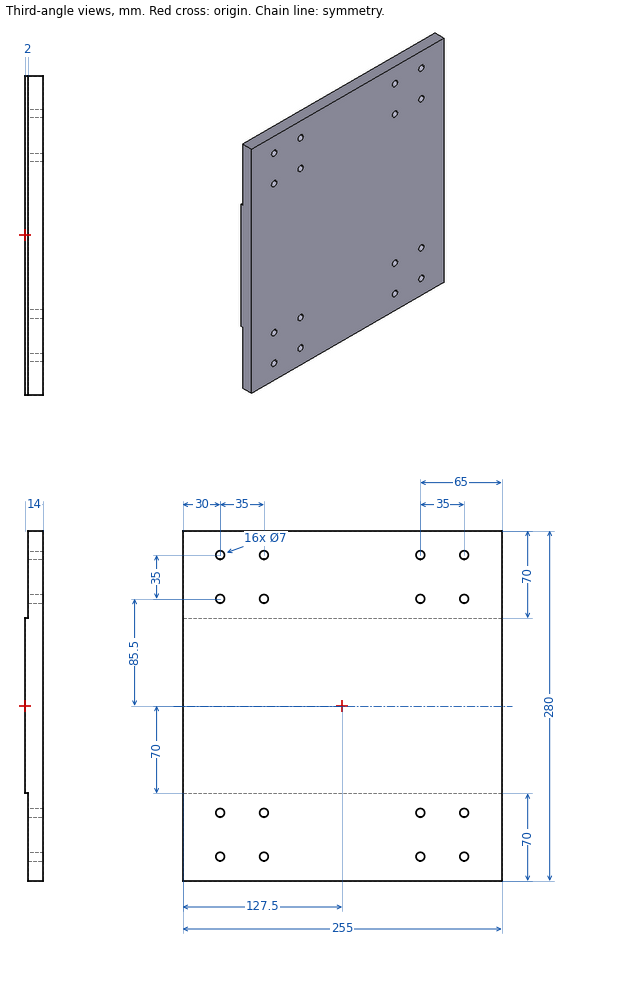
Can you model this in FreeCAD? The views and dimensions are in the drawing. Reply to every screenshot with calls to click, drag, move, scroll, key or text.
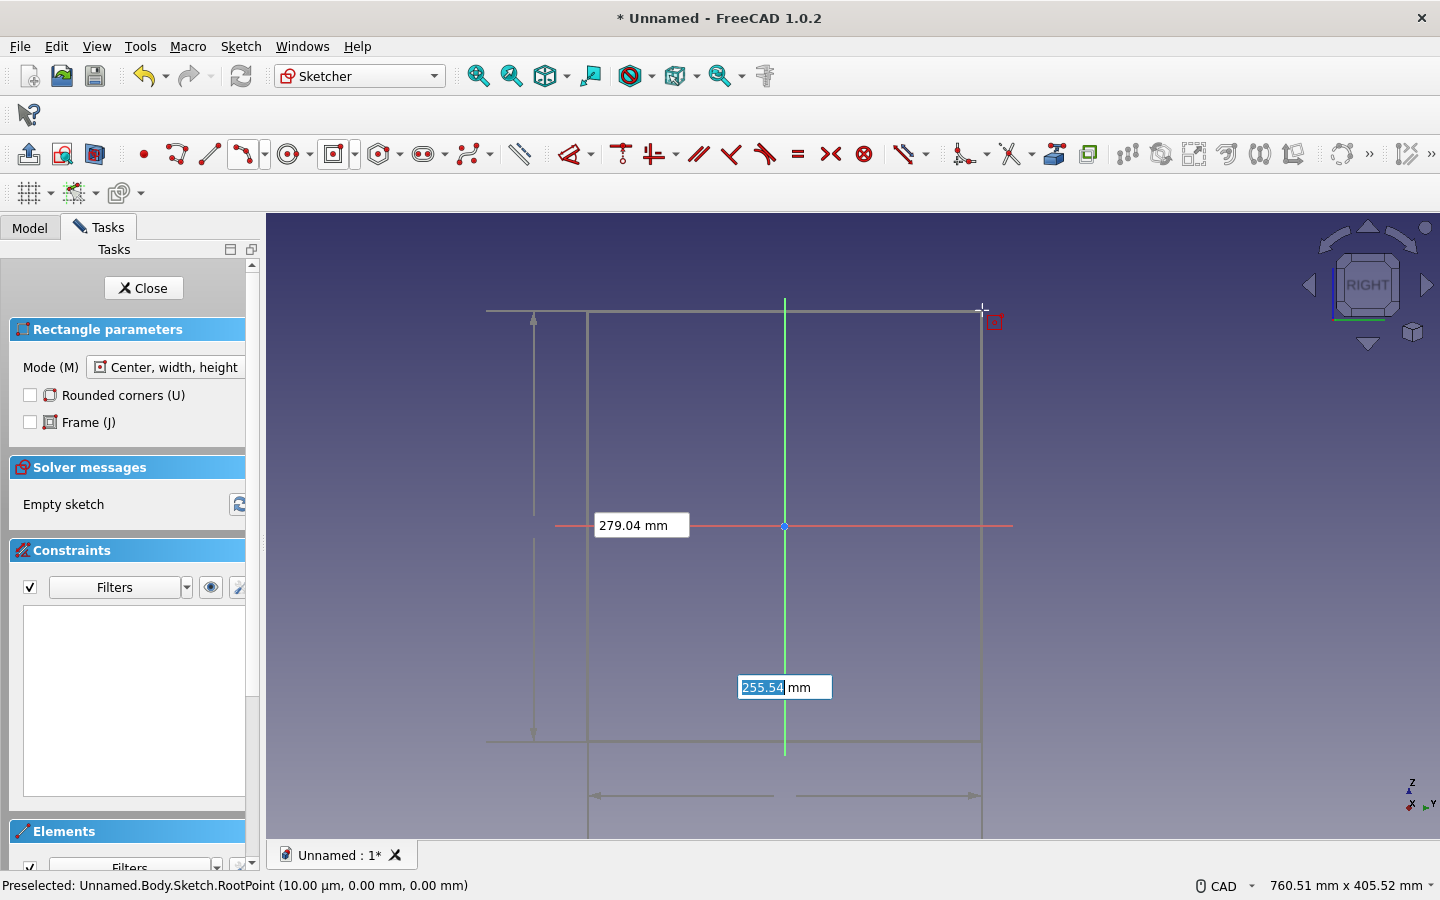
text(255)
key(Tab)
text(280)
key(Return)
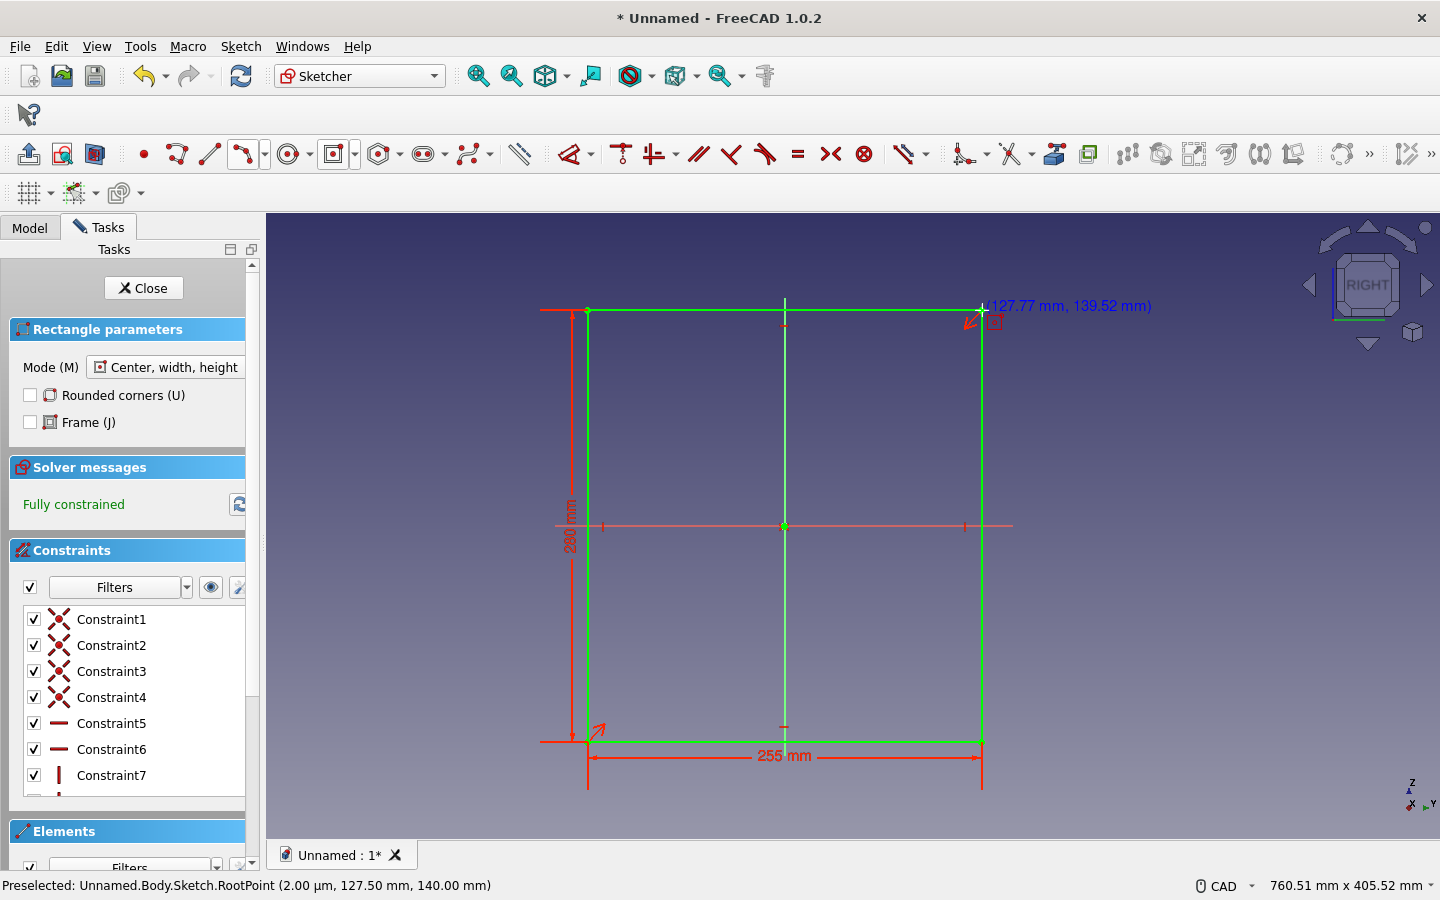
click(288, 154)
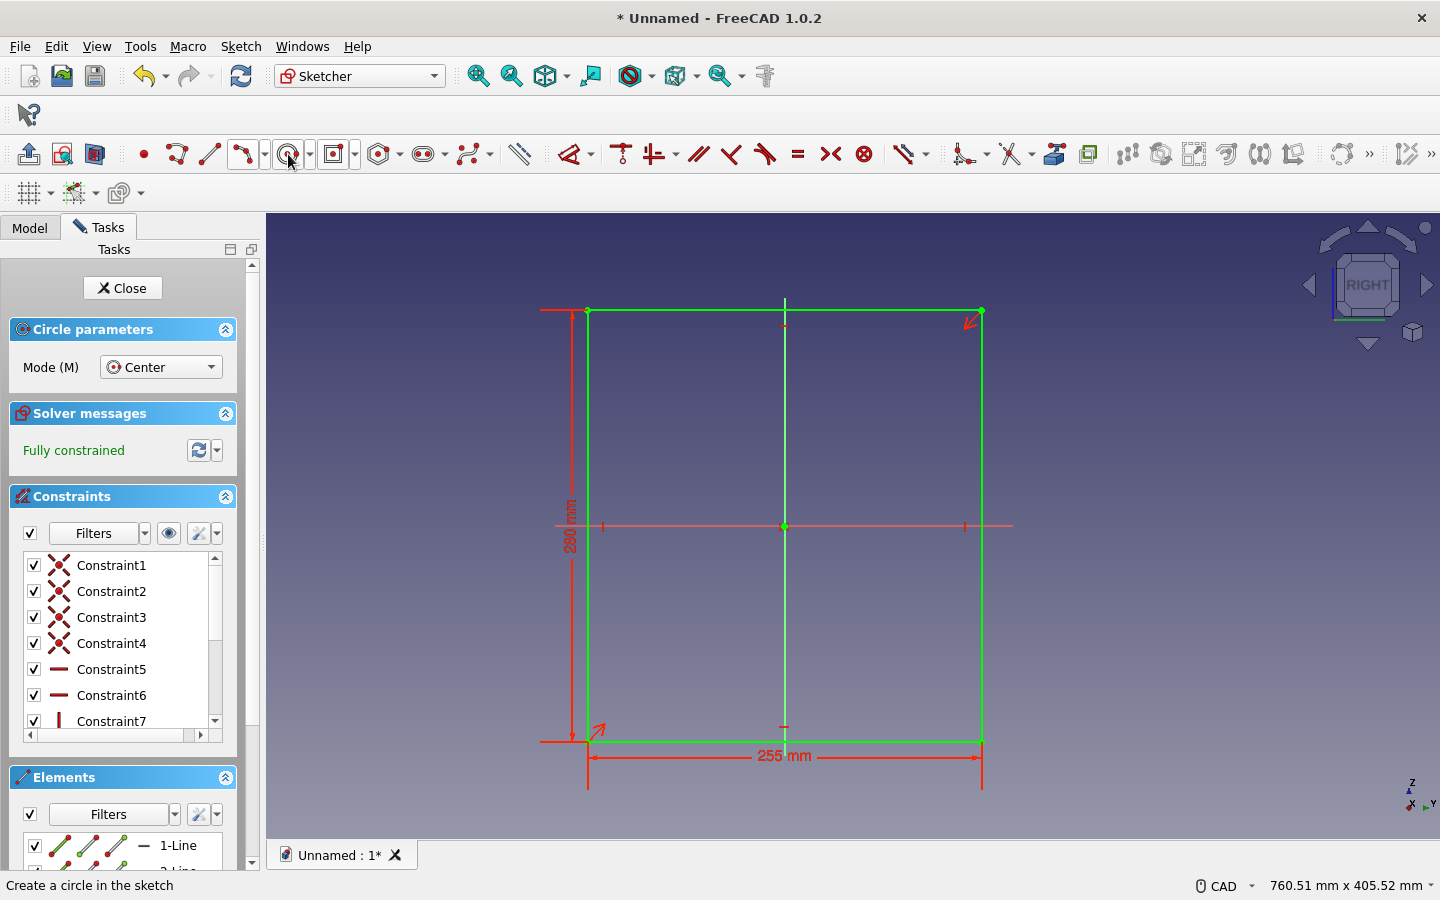
scroll(634, 340, up, 8)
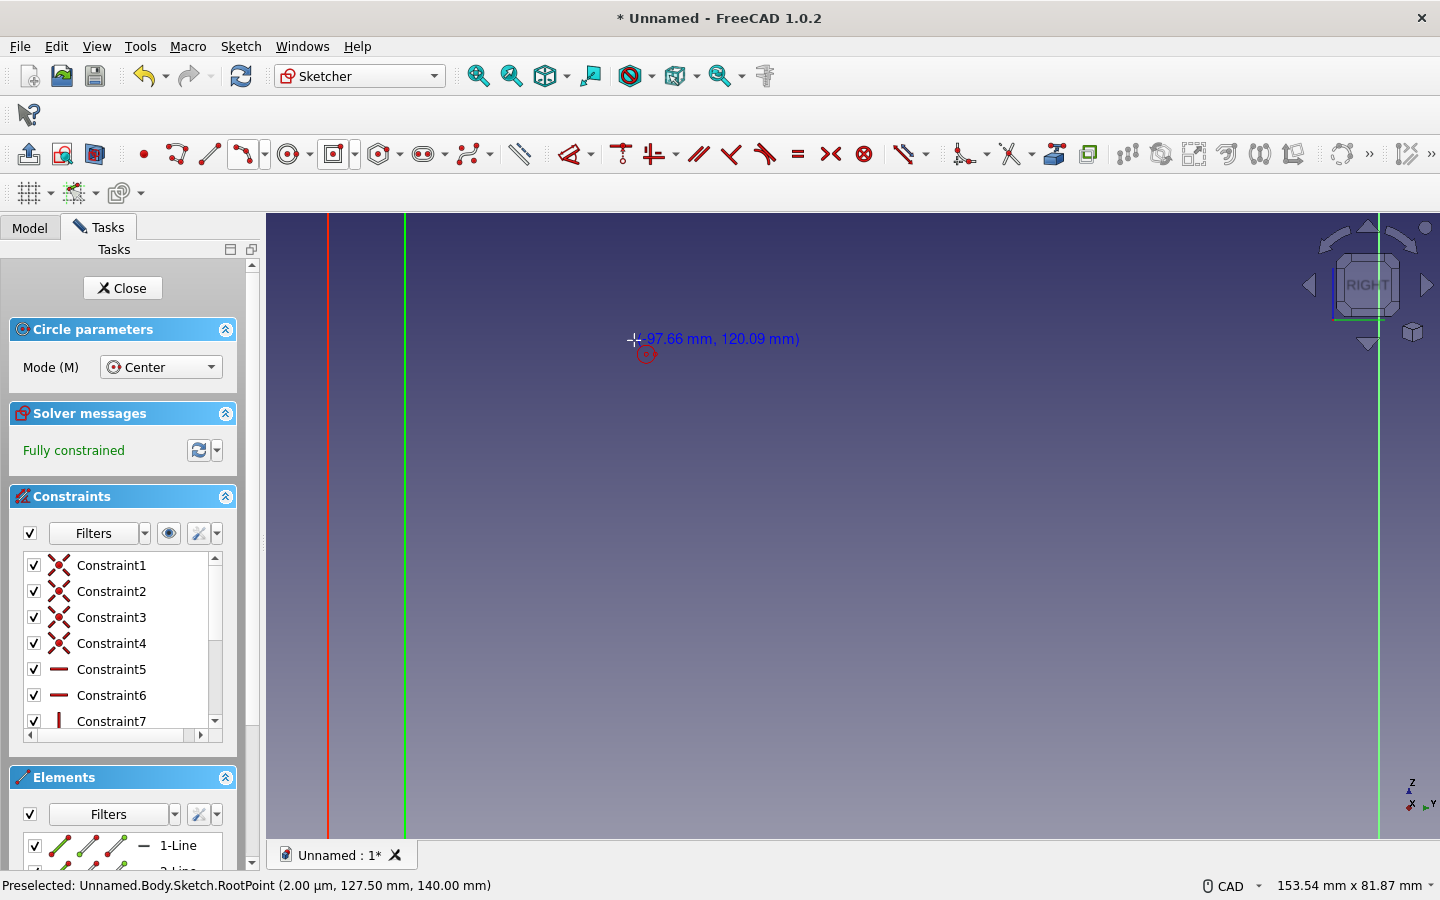
scroll(634, 340, down, 8)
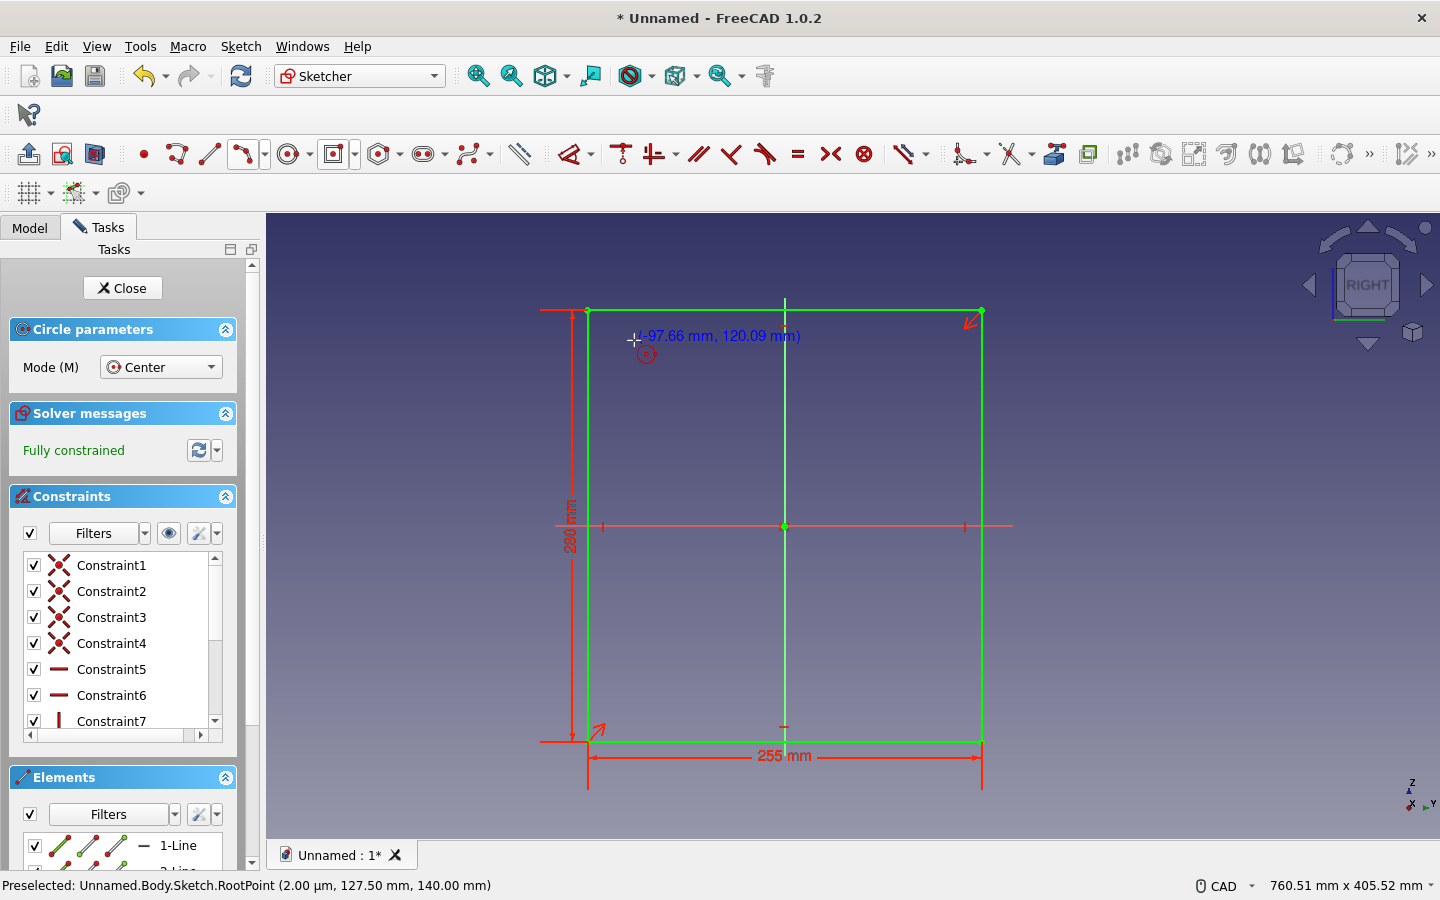
click(634, 340)
move(638, 337)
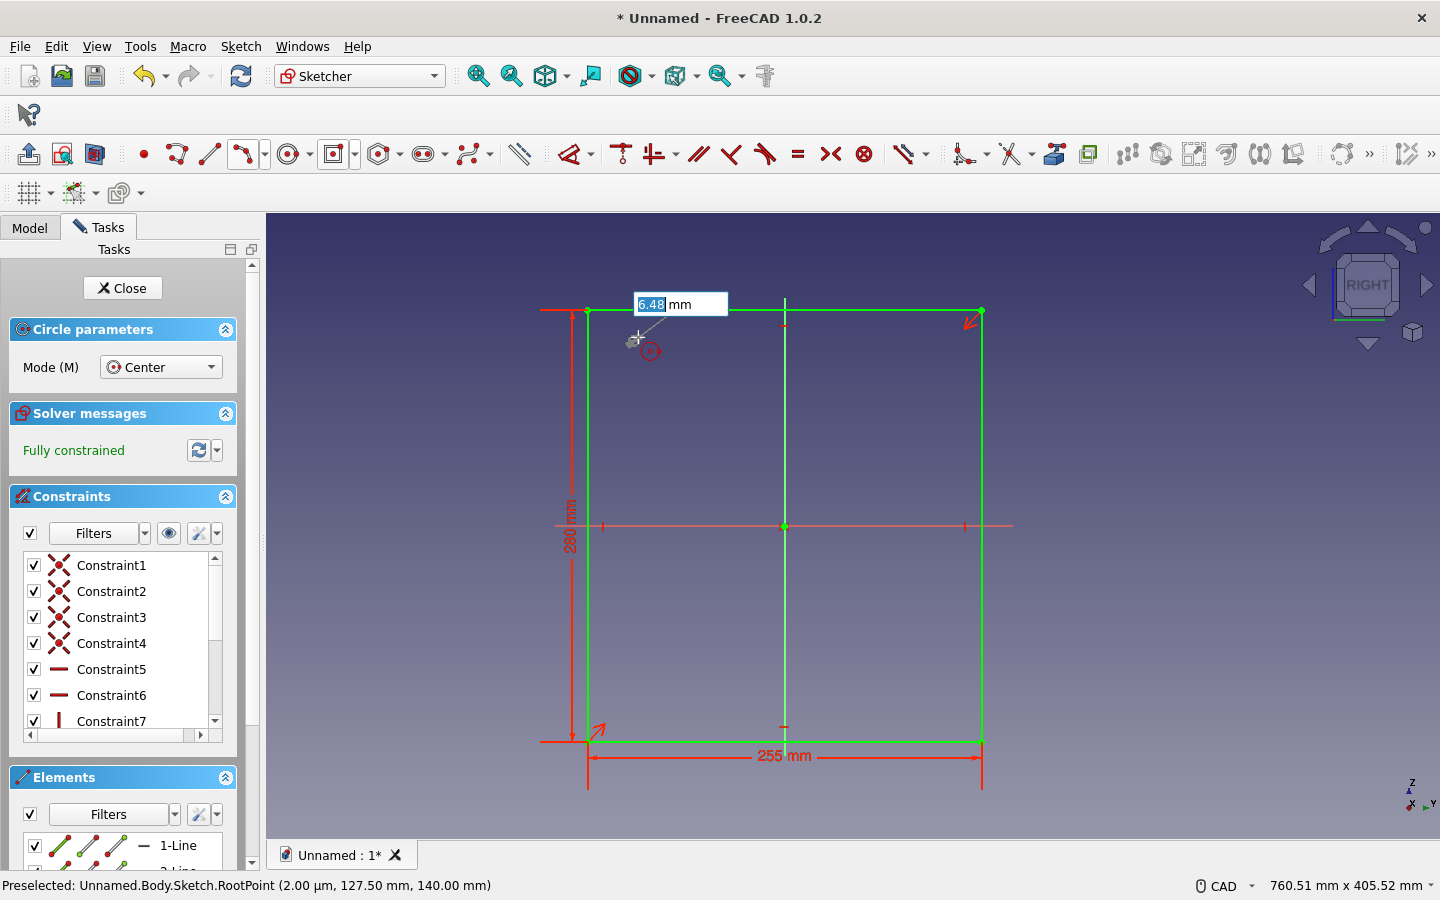
text(7)
key(Return)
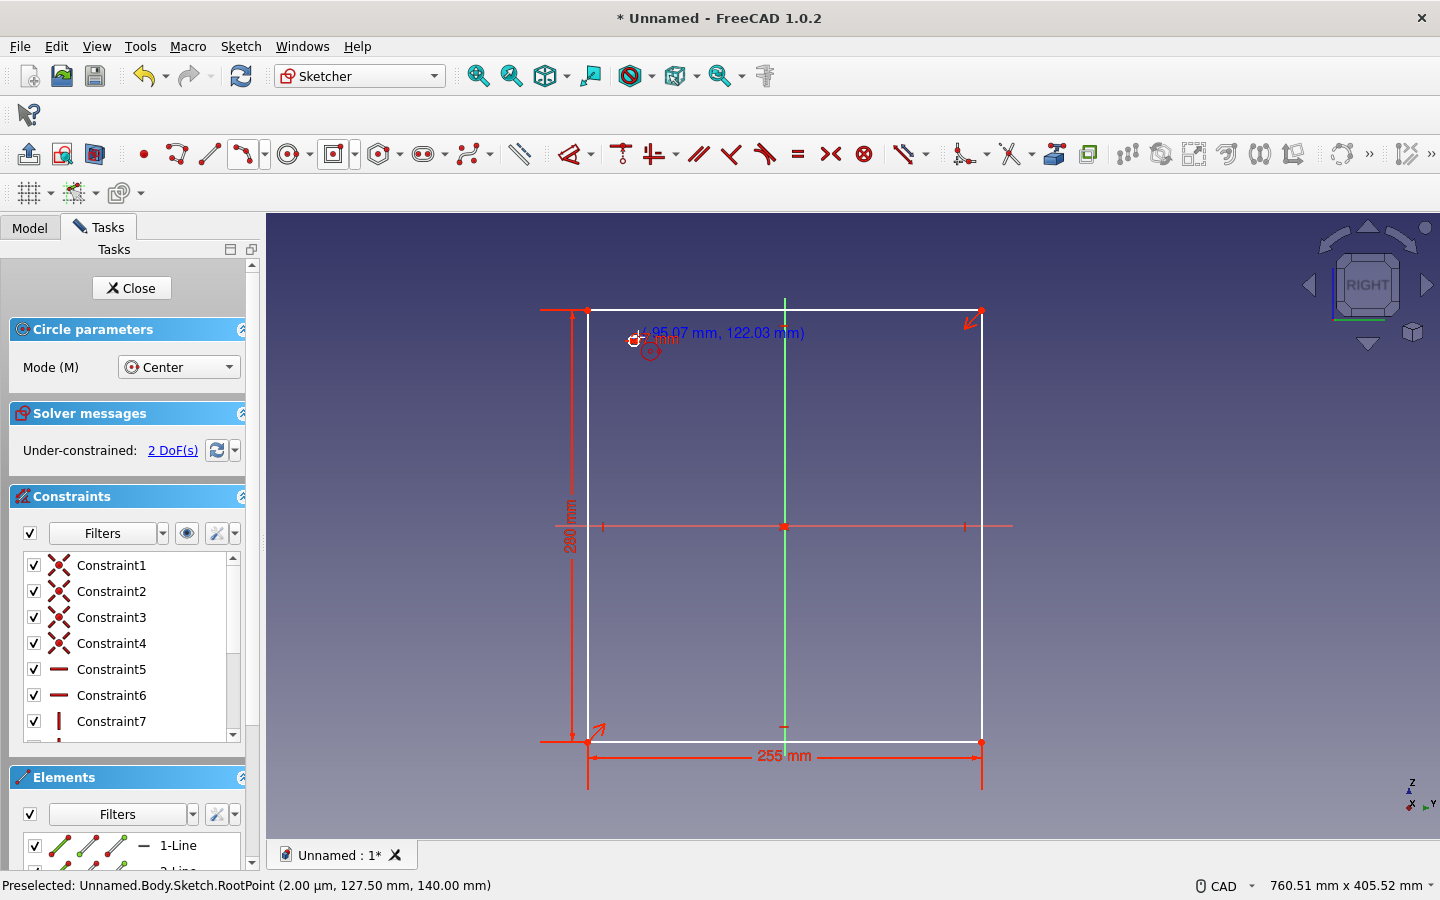
scroll(634, 394, up, 8)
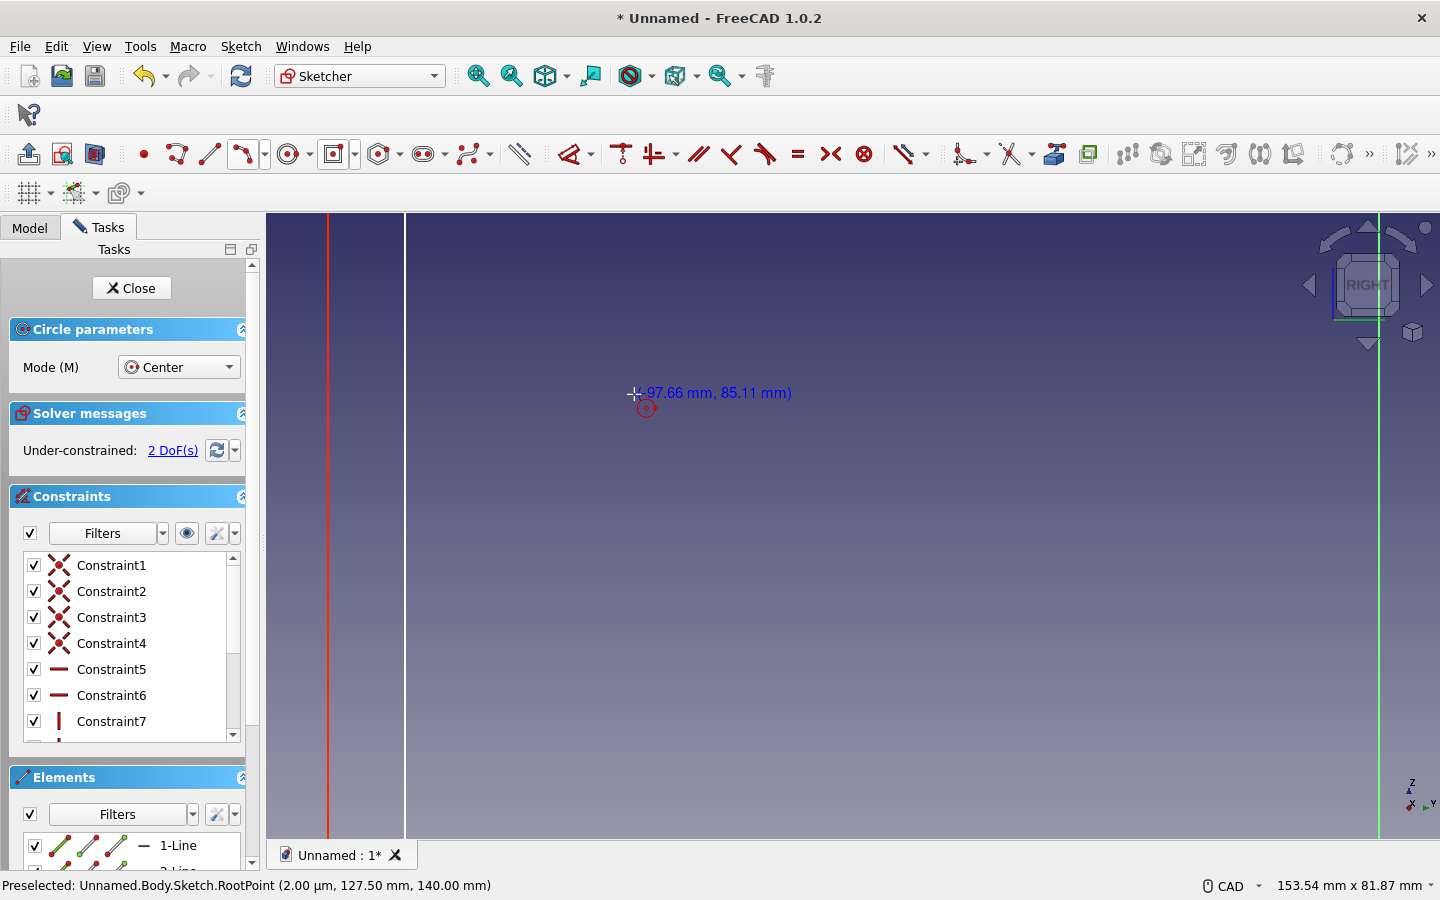
scroll(634, 394, down, 8)